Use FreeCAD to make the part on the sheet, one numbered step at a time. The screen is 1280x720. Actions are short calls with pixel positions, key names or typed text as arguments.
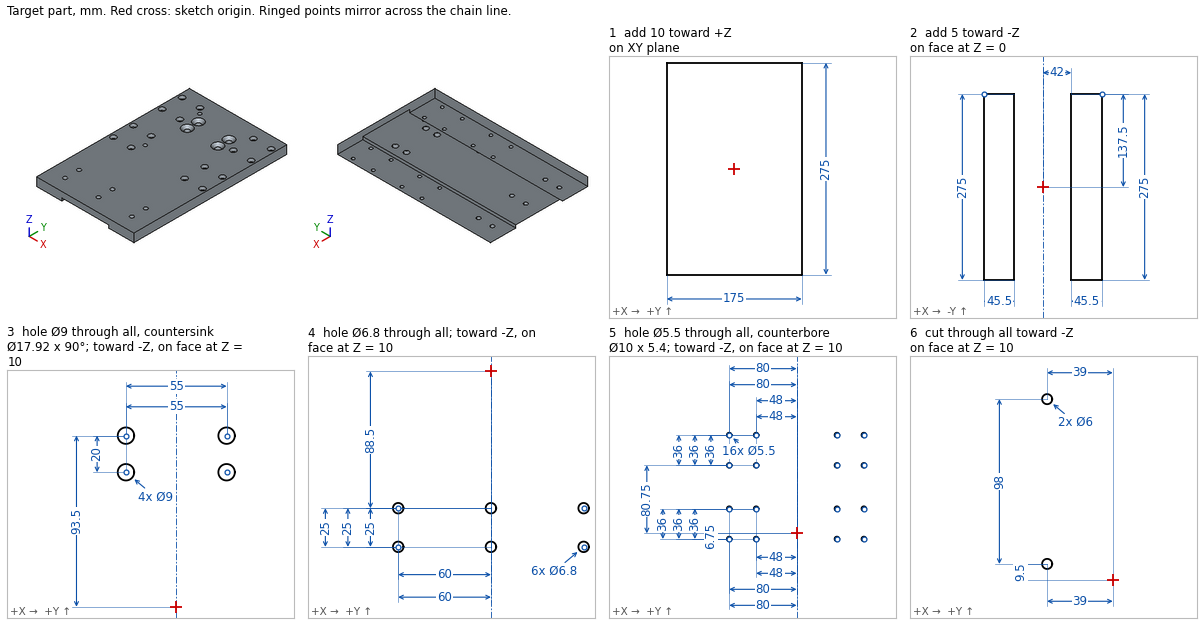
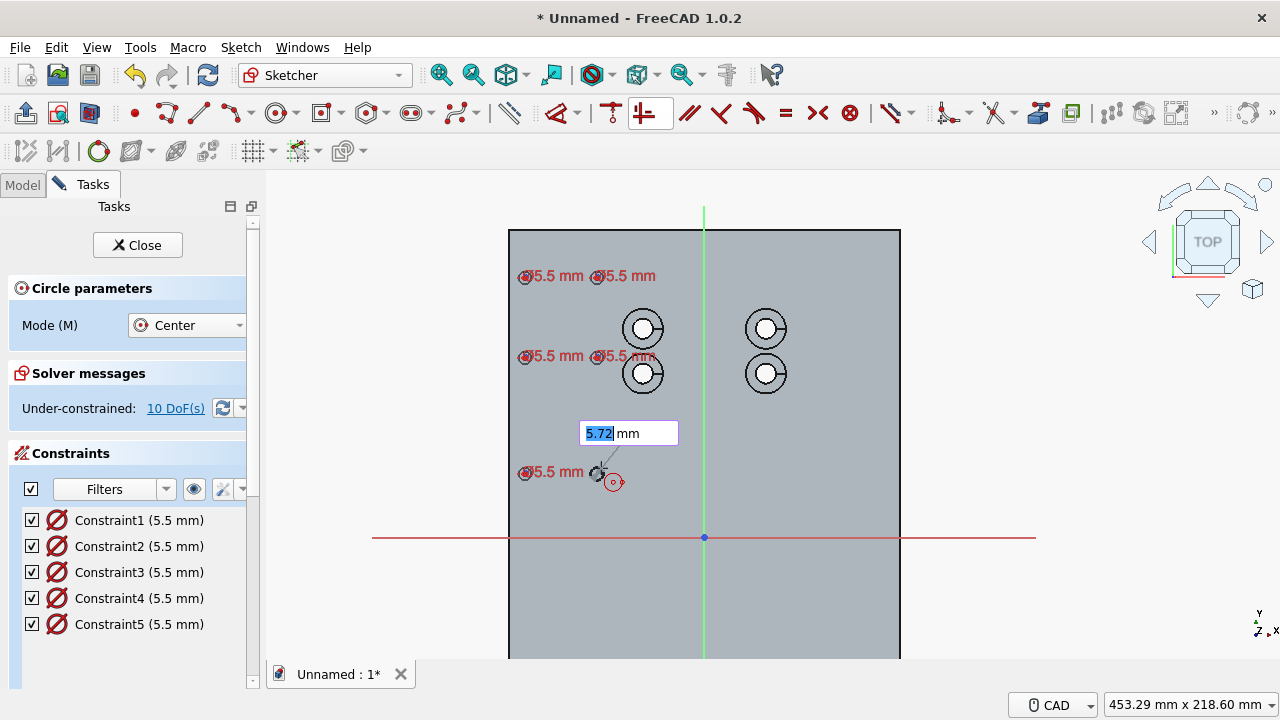
text(5.5)
key(Return)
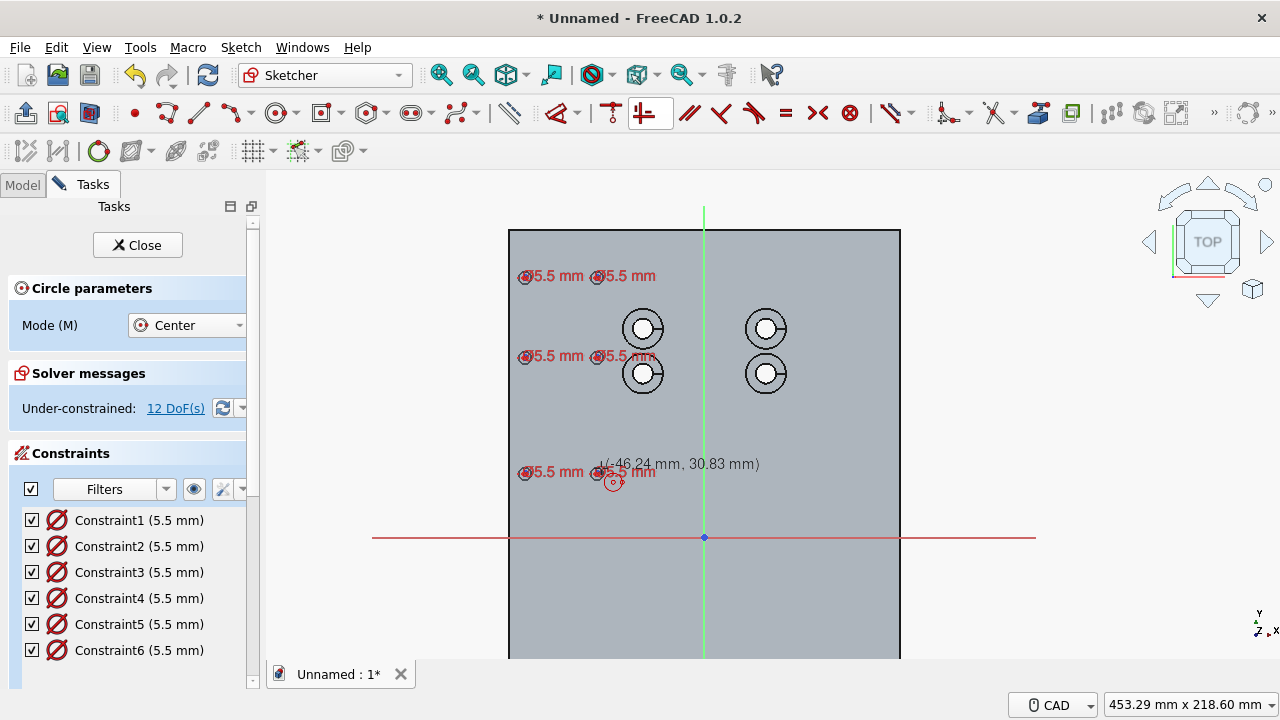
scroll(525, 553, up, 7)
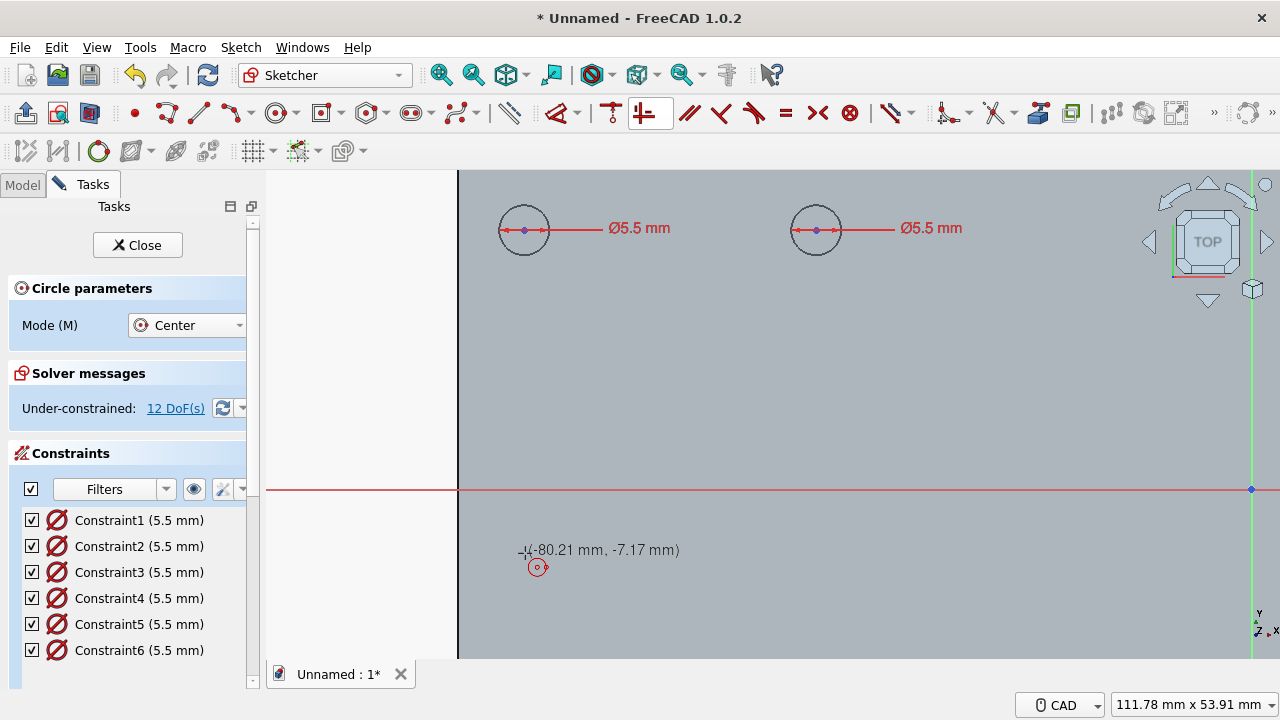
scroll(525, 553, down, 7)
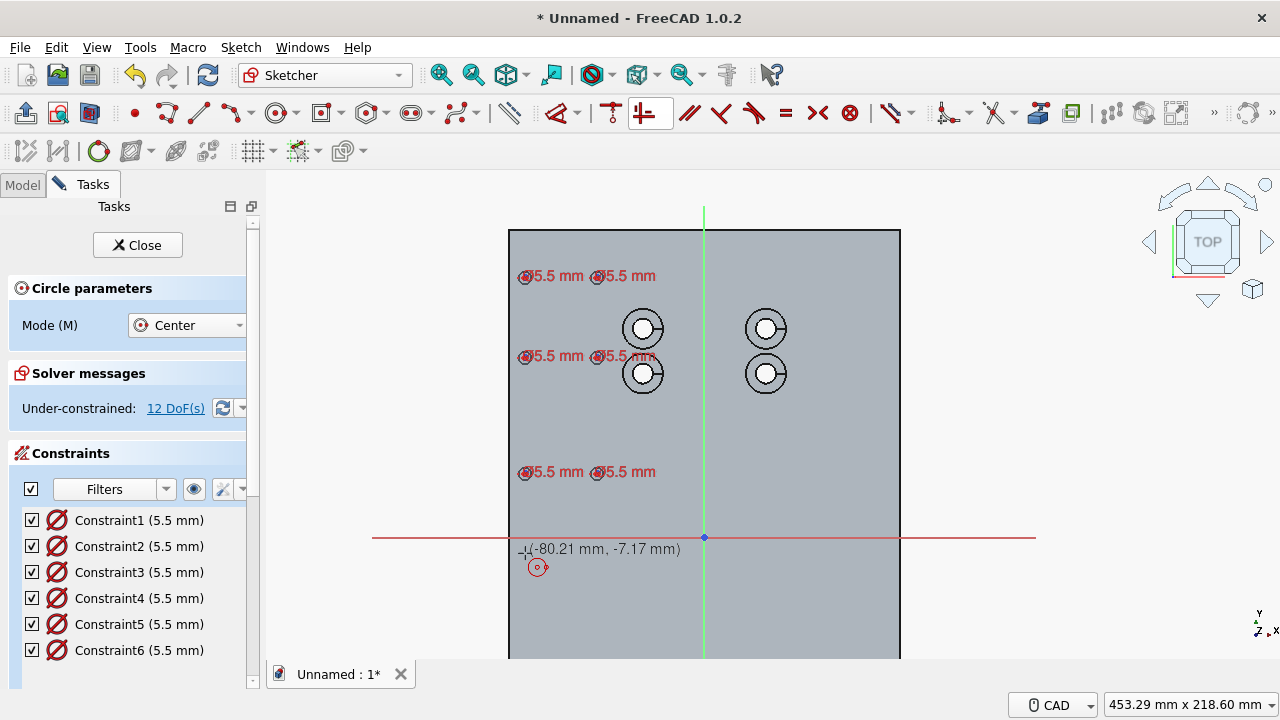
click(525, 553)
move(530, 557)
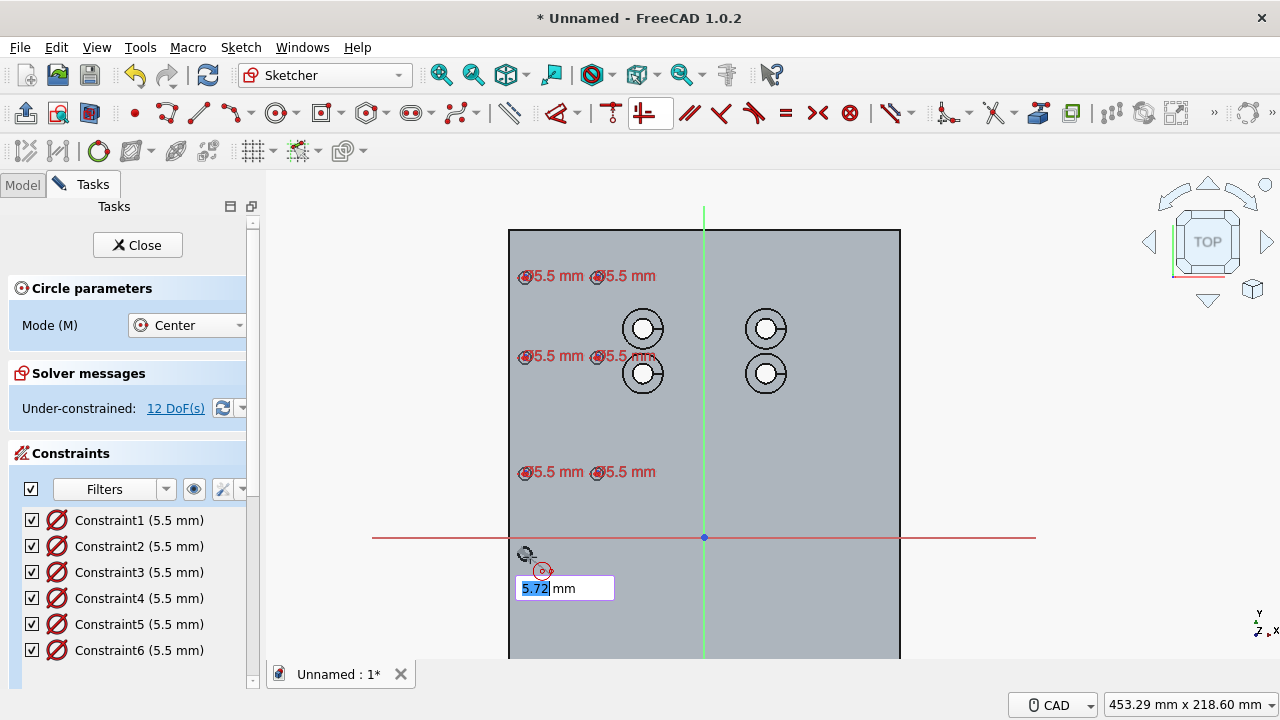
text(5.5)
key(Return)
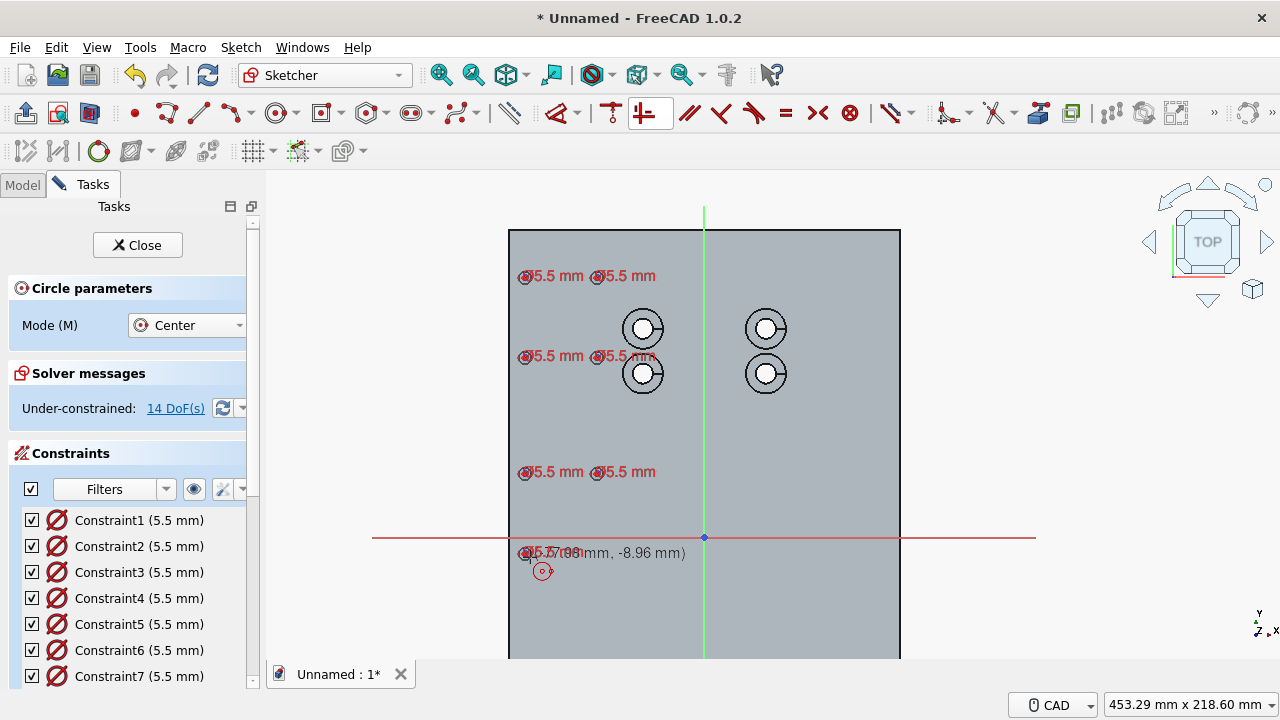
scroll(597, 553, up, 7)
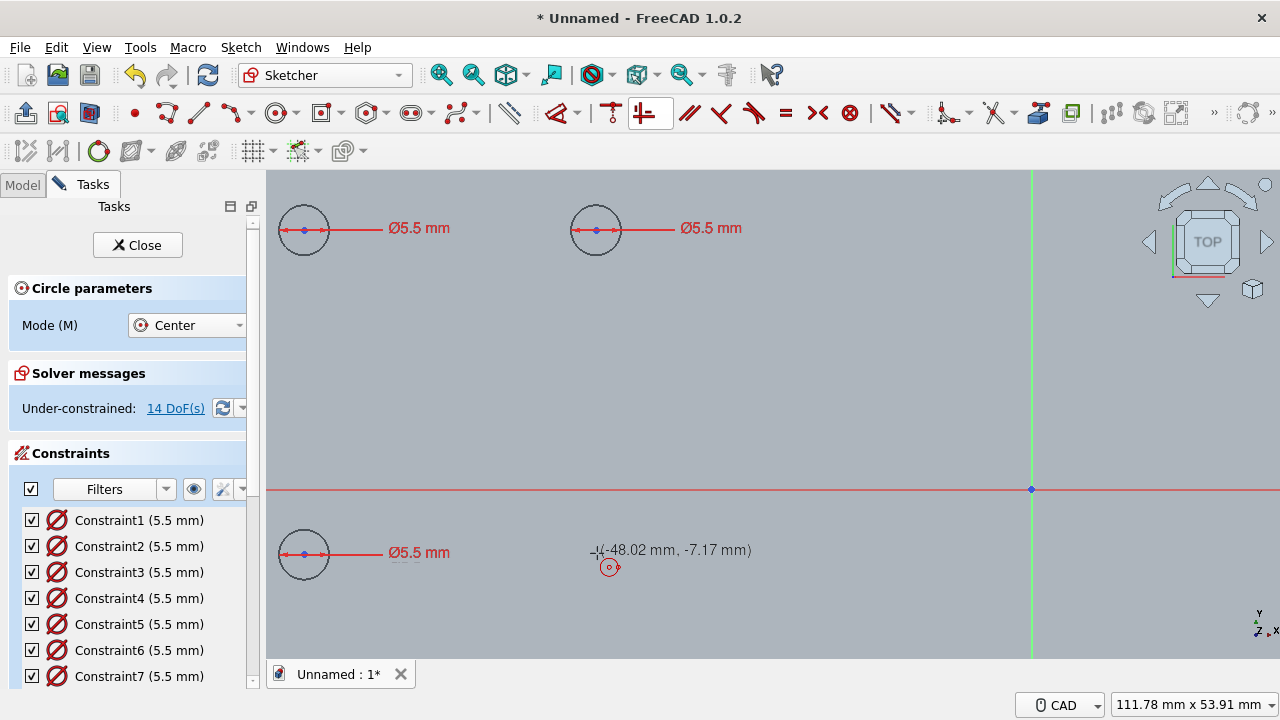
scroll(597, 553, down, 7)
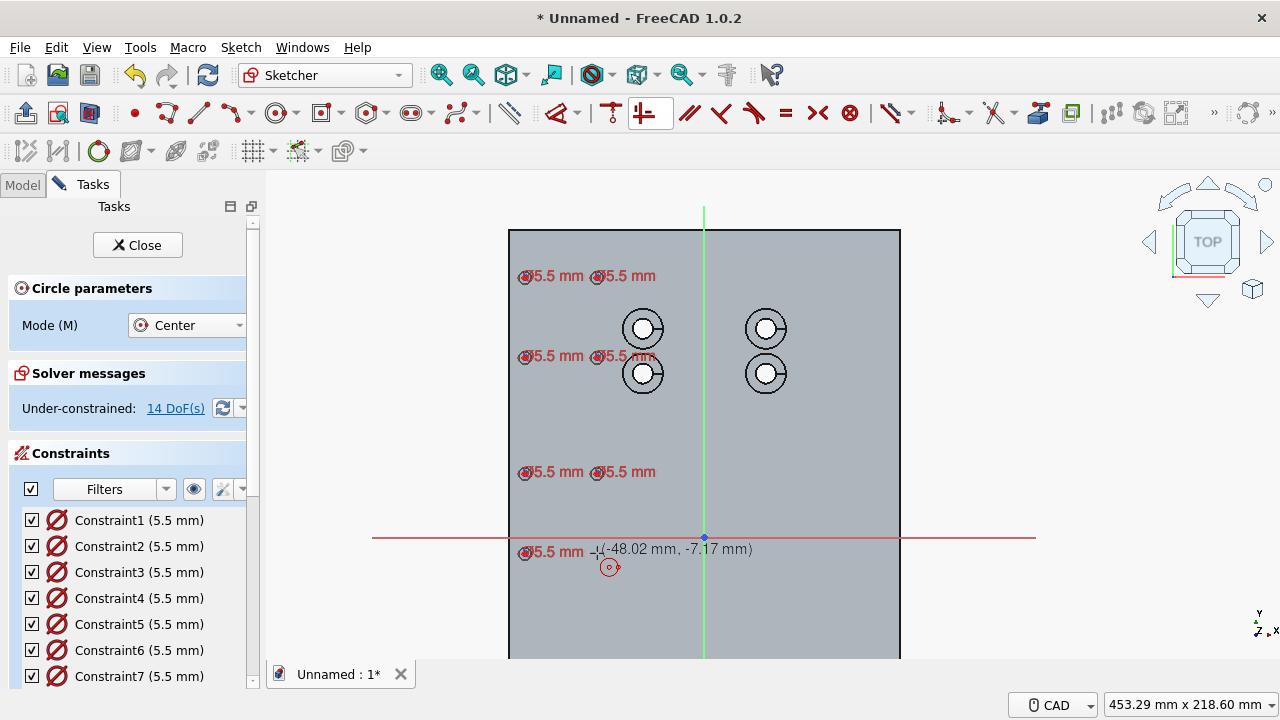
click(597, 553)
move(601, 557)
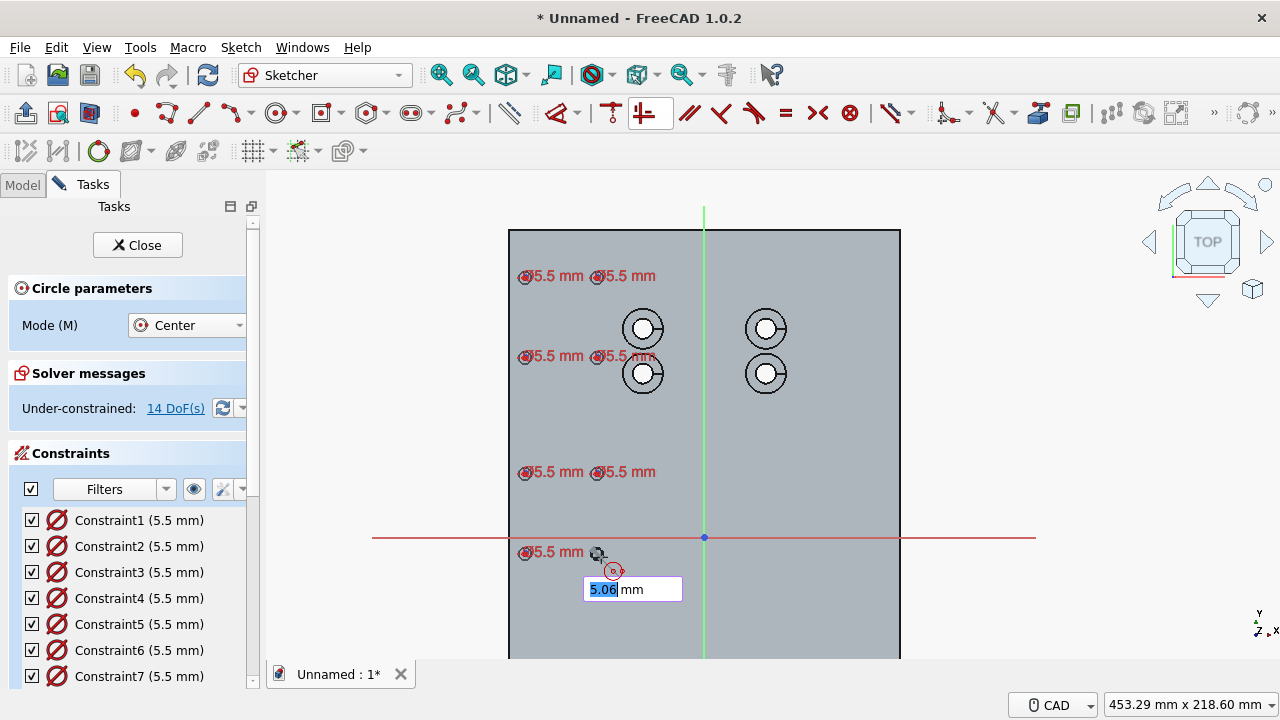
text(5.5)
key(Return)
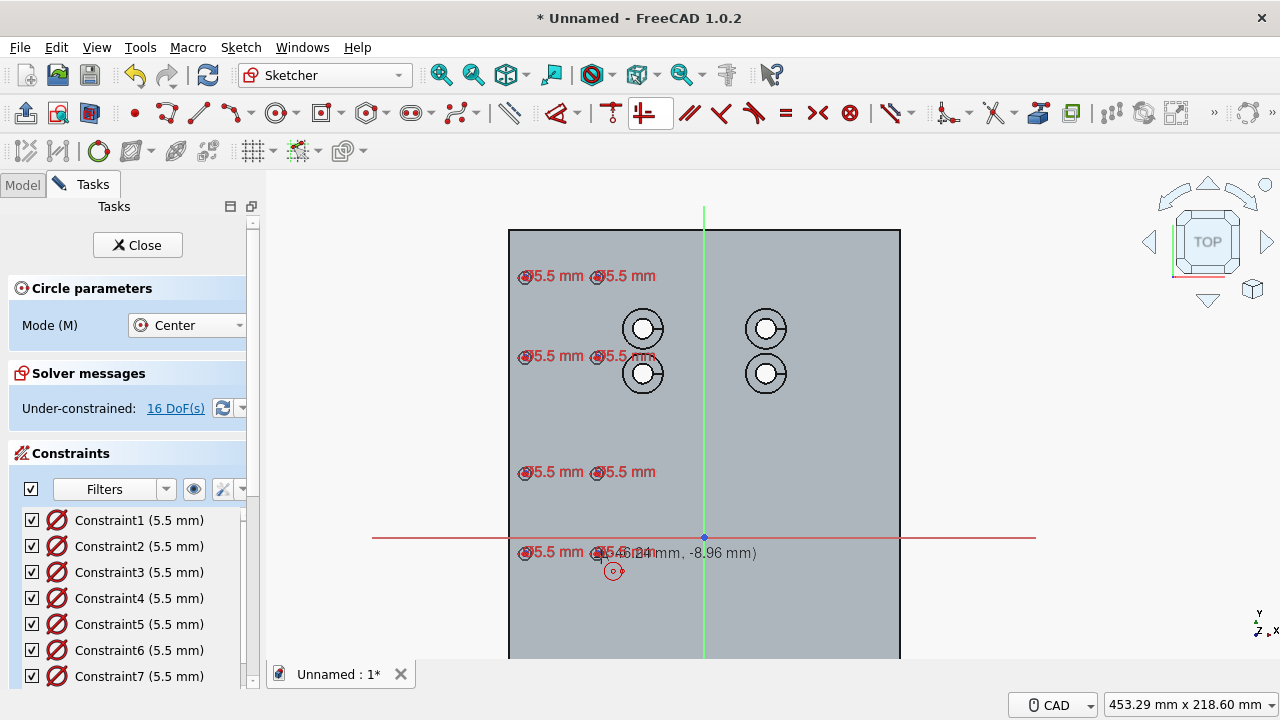
scroll(812, 553, up, 7)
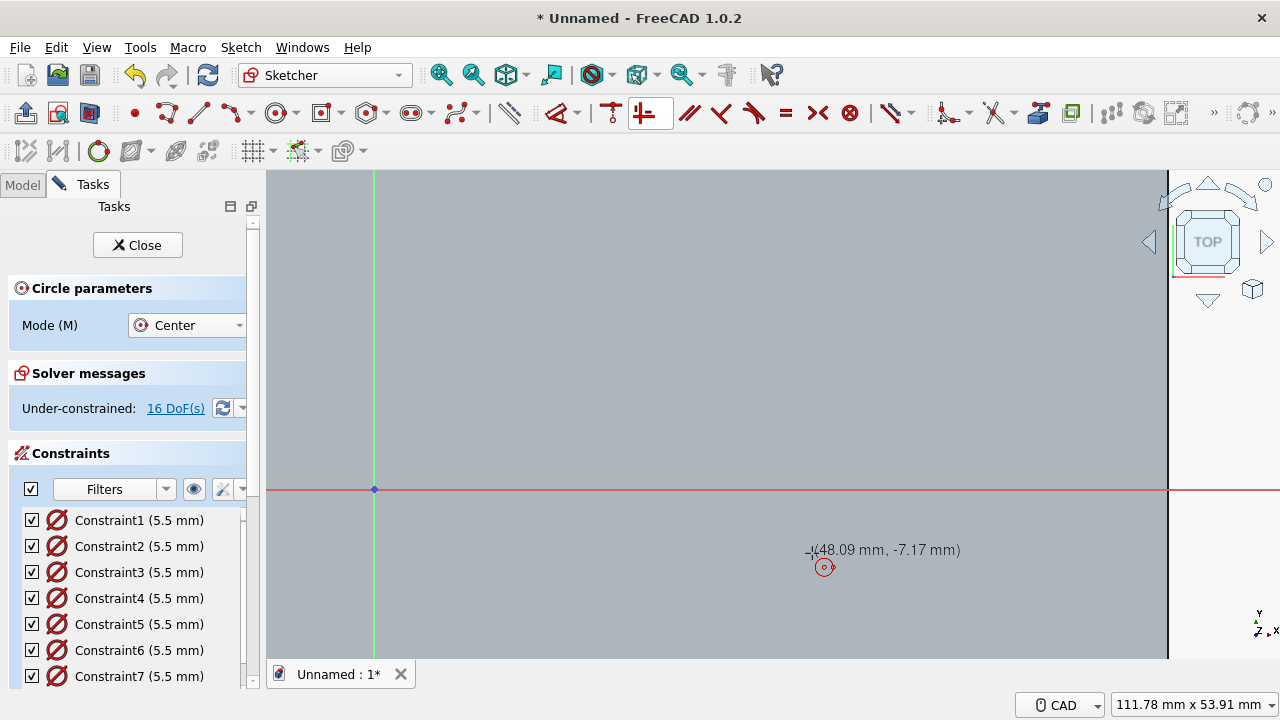
scroll(813, 553, down, 7)